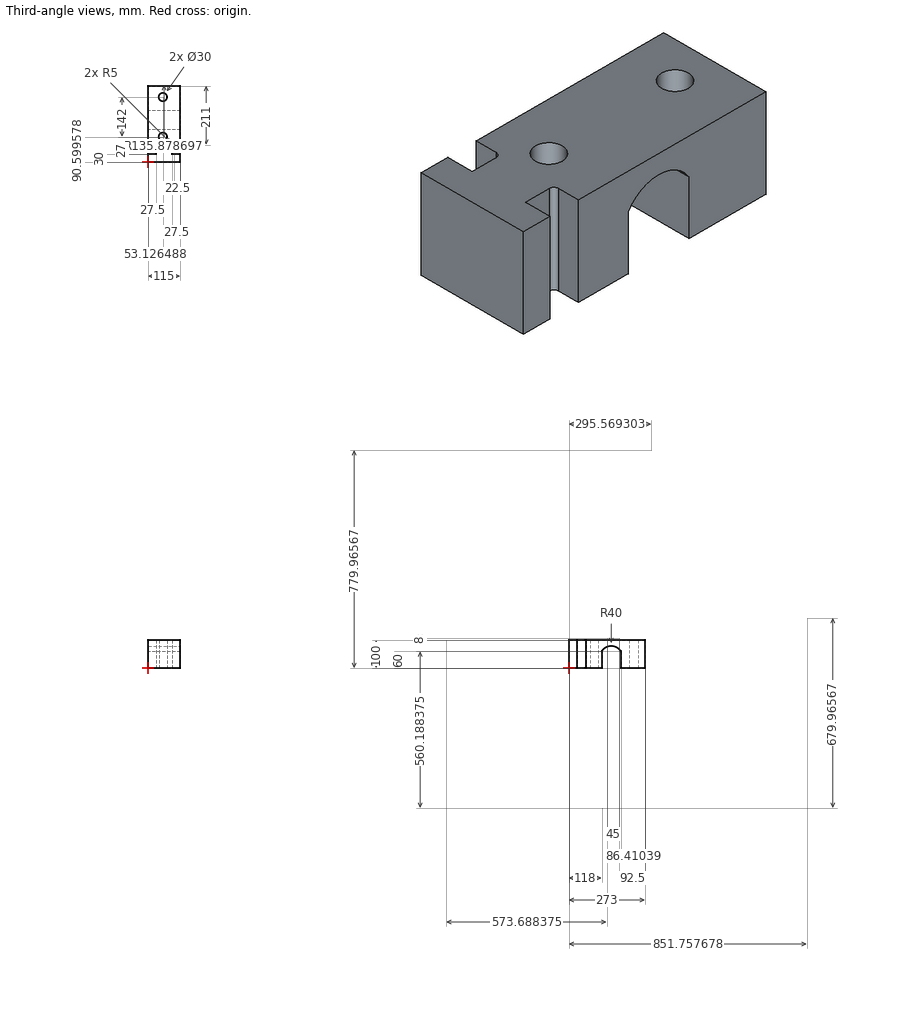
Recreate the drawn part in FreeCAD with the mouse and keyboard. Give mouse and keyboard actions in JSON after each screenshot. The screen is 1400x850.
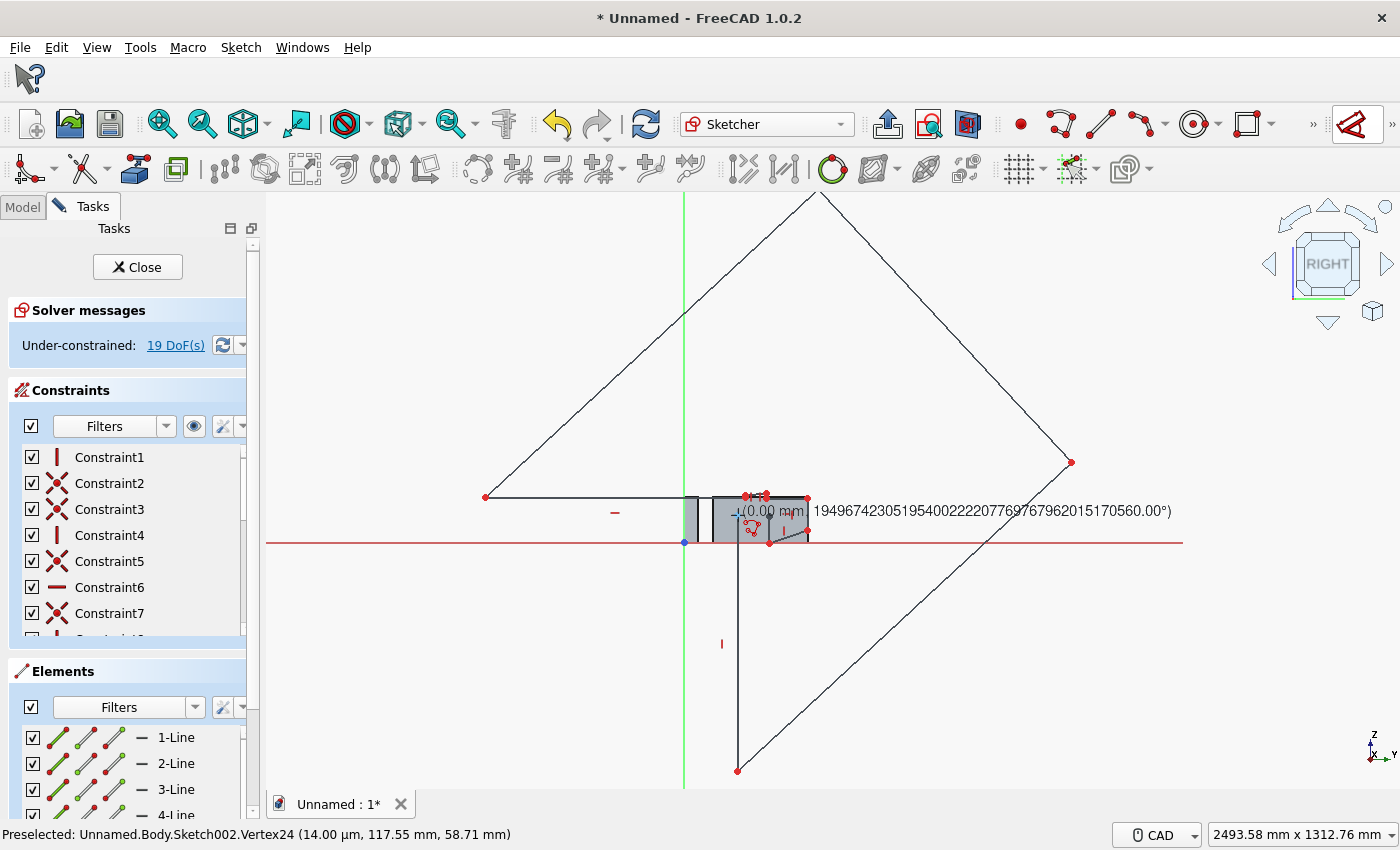
{"action": "key", "text": "g 3 a"}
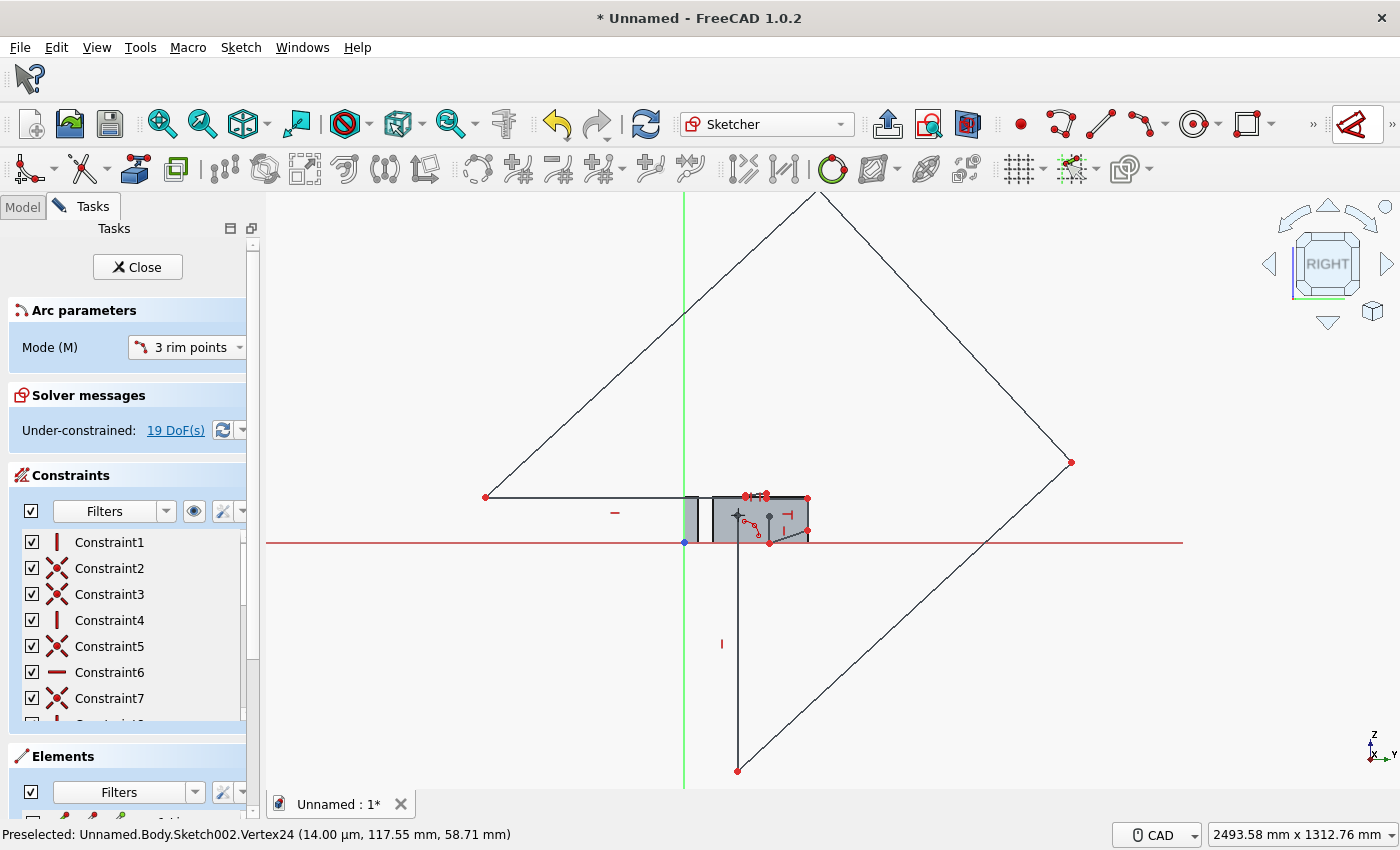
{"action": "left_click", "coordinate": [738, 516]}
{"action": "left_click", "coordinate": [769, 517]}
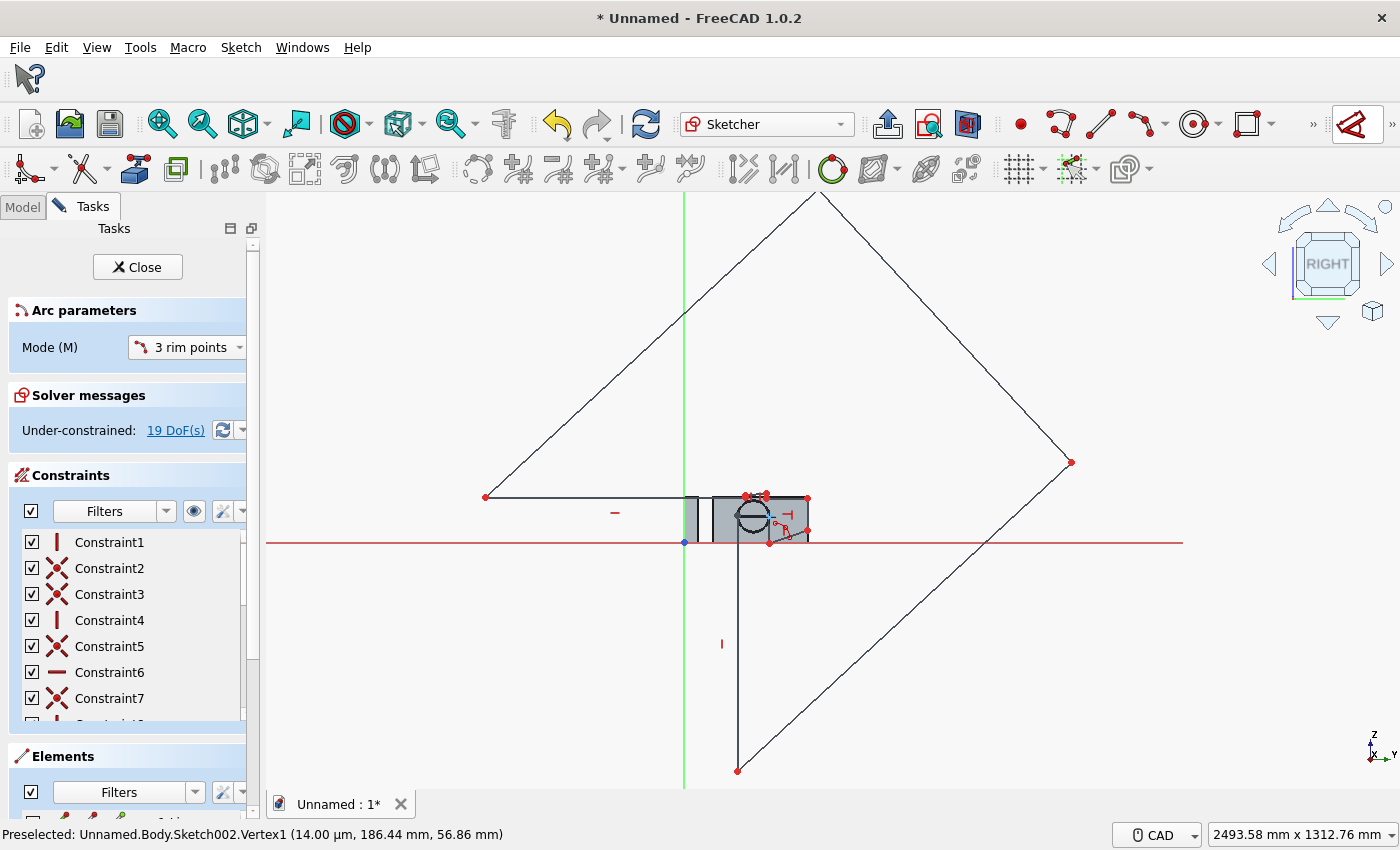
{"action": "scroll", "coordinate": [754, 507], "scroll_direction": "up", "scroll_amount": 3}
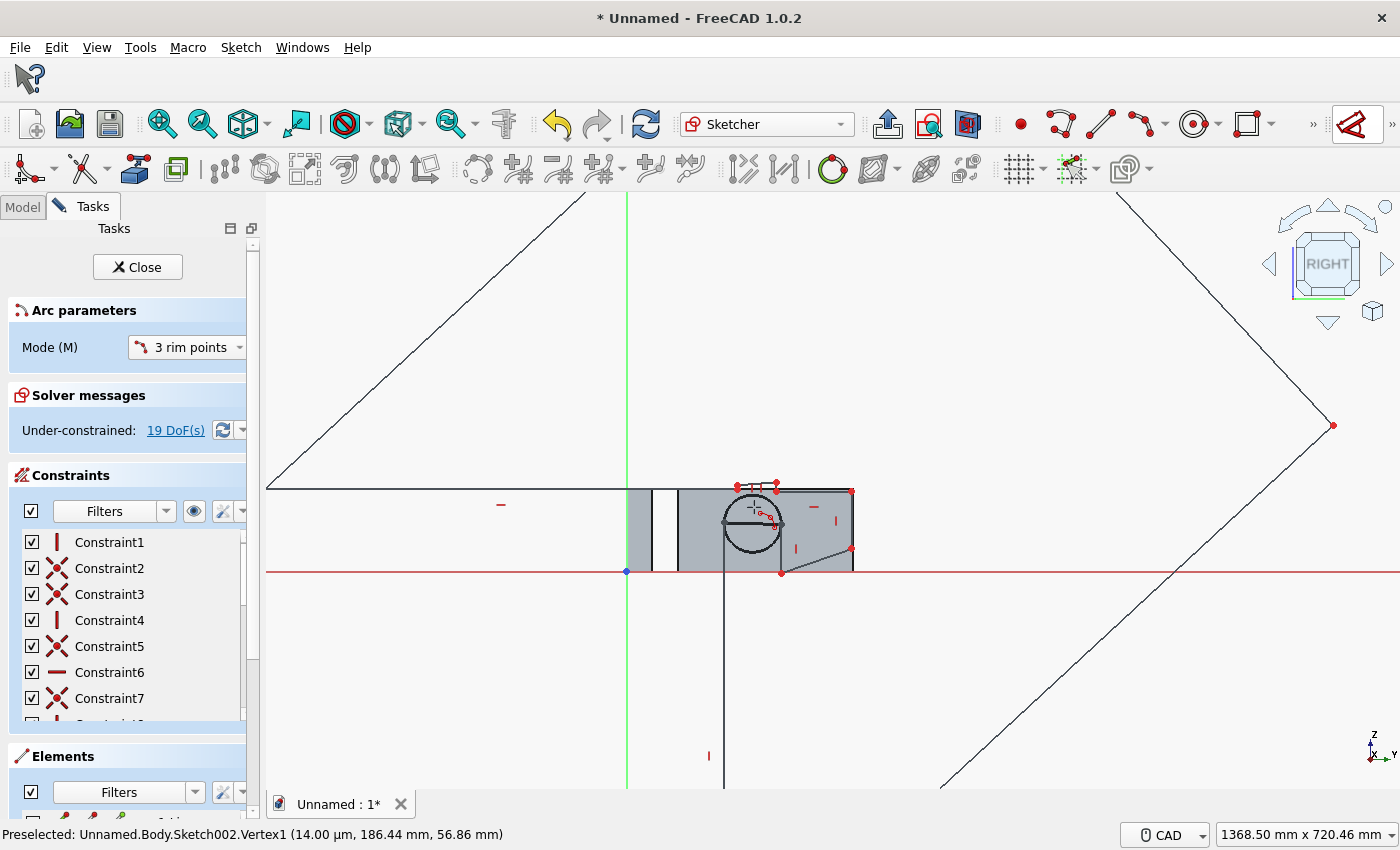
{"action": "left_click", "coordinate": [753, 506]}
{"action": "key", "text": "Escape"}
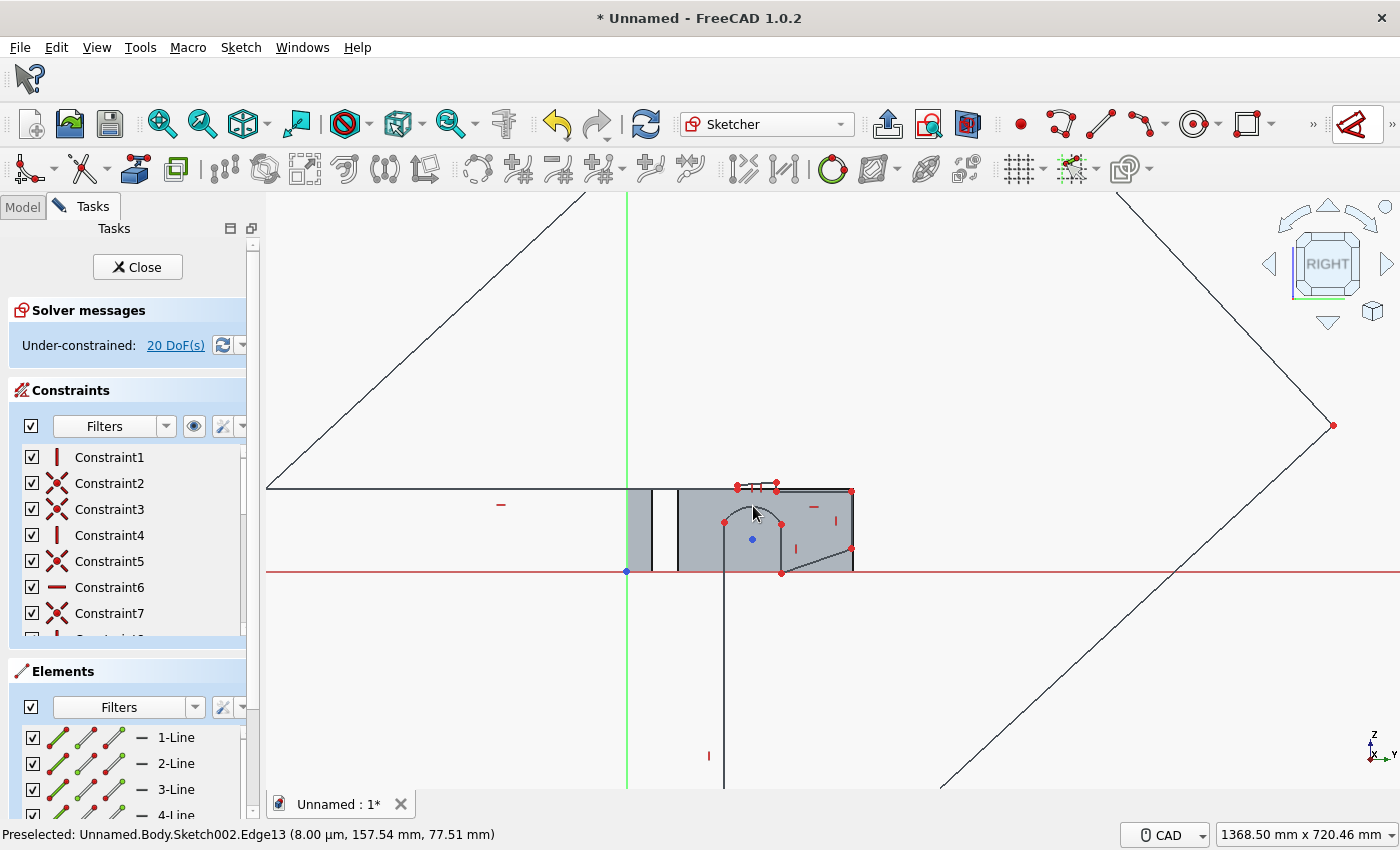
{"action": "left_click", "coordinate": [831, 556]}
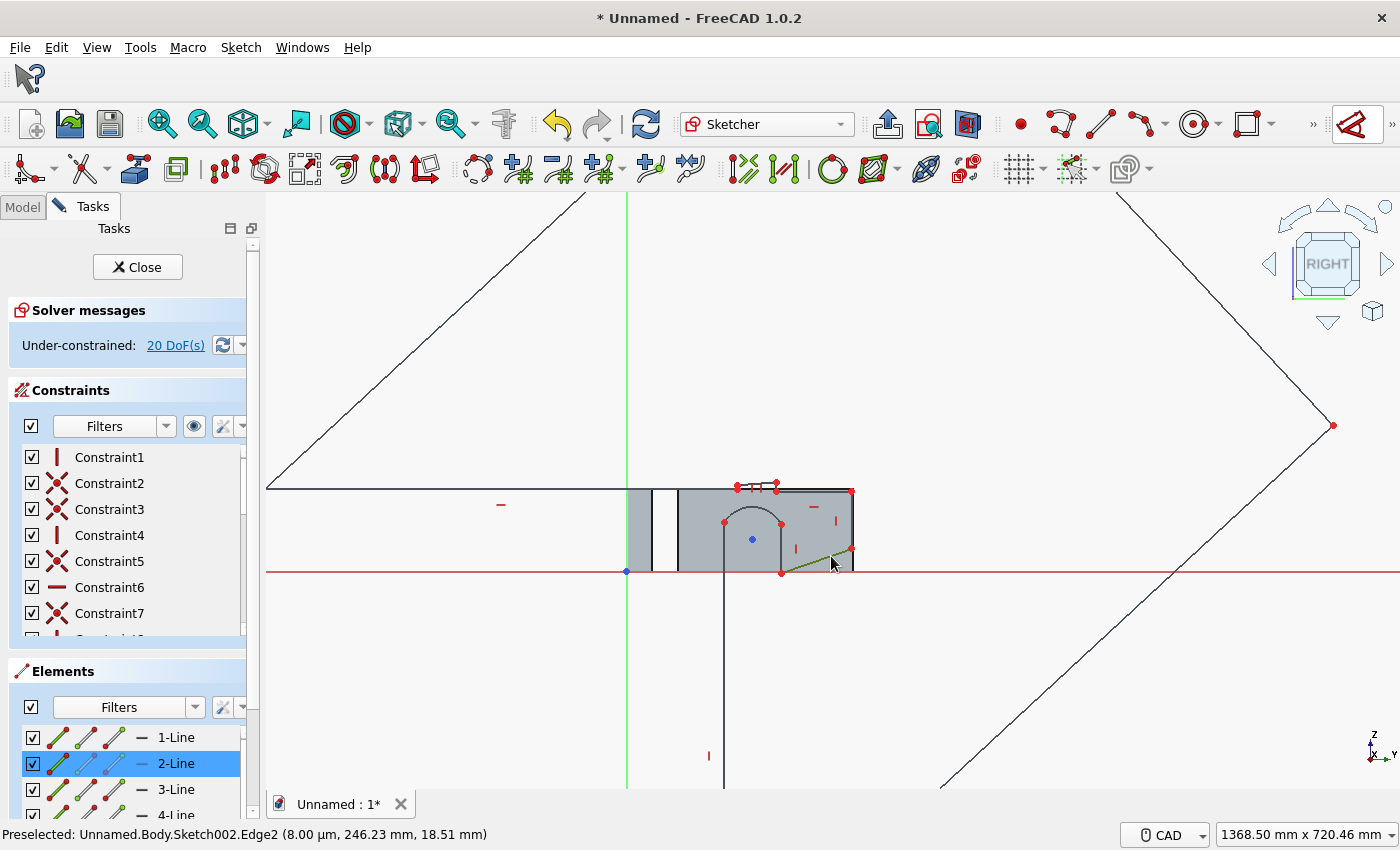
{"action": "key", "text": "h"}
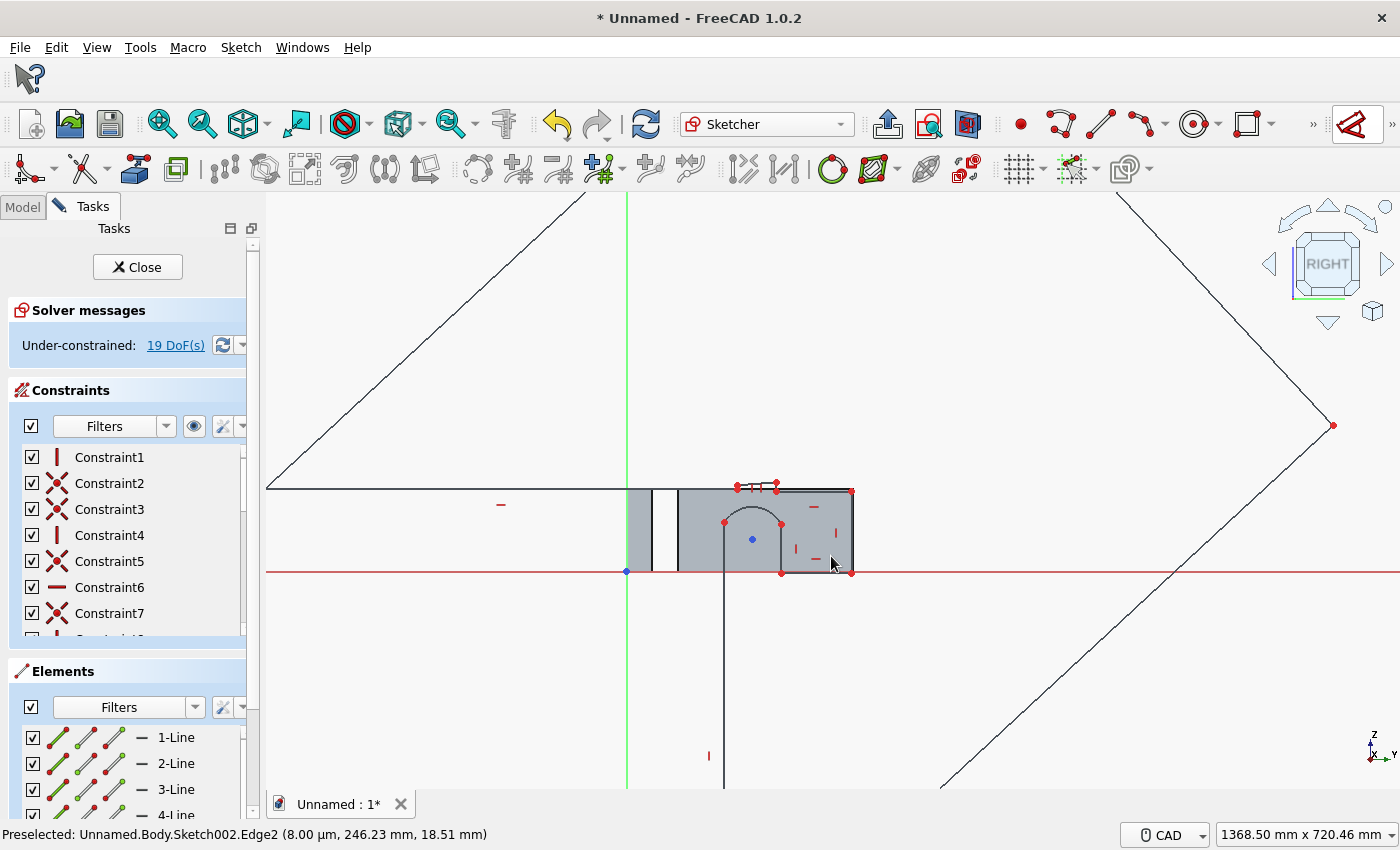
{"action": "left_click", "coordinate": [745, 485]}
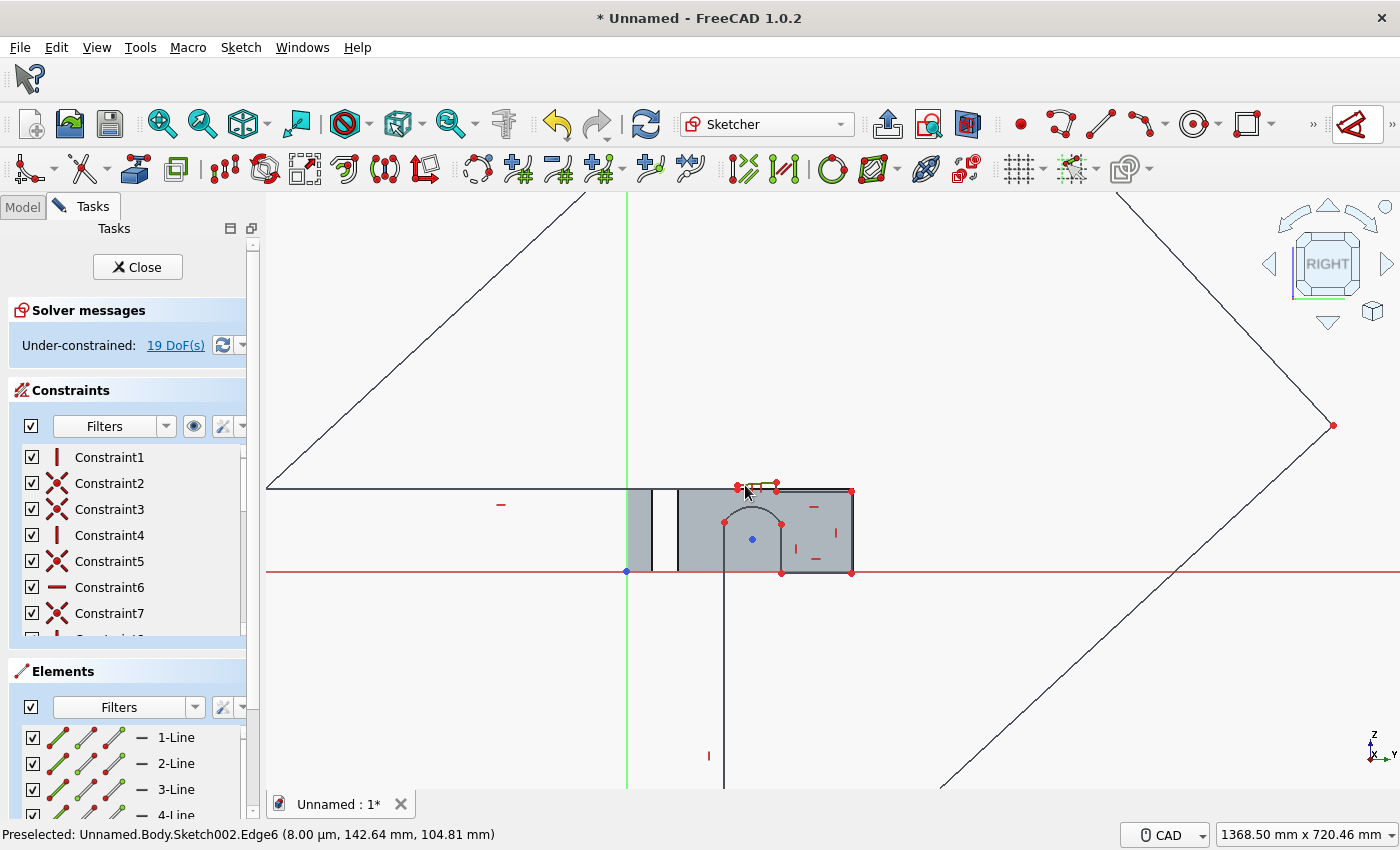
{"action": "key", "text": "h"}